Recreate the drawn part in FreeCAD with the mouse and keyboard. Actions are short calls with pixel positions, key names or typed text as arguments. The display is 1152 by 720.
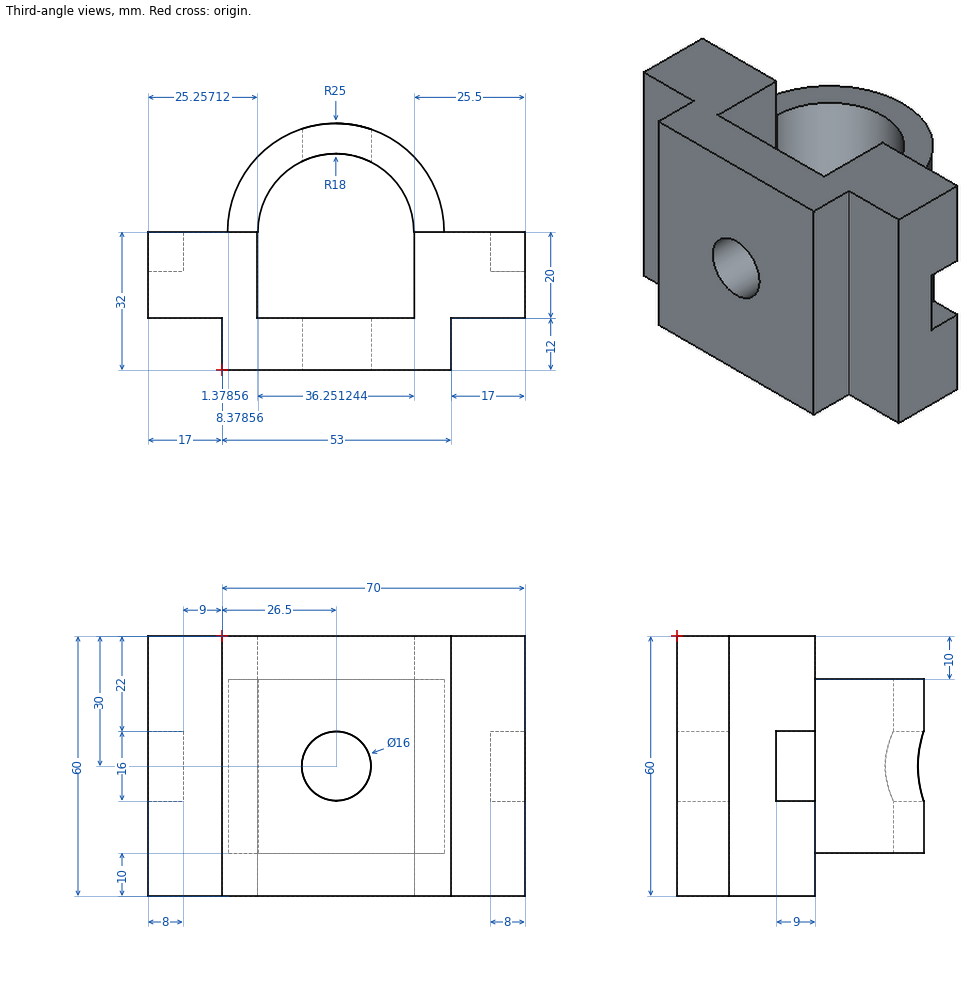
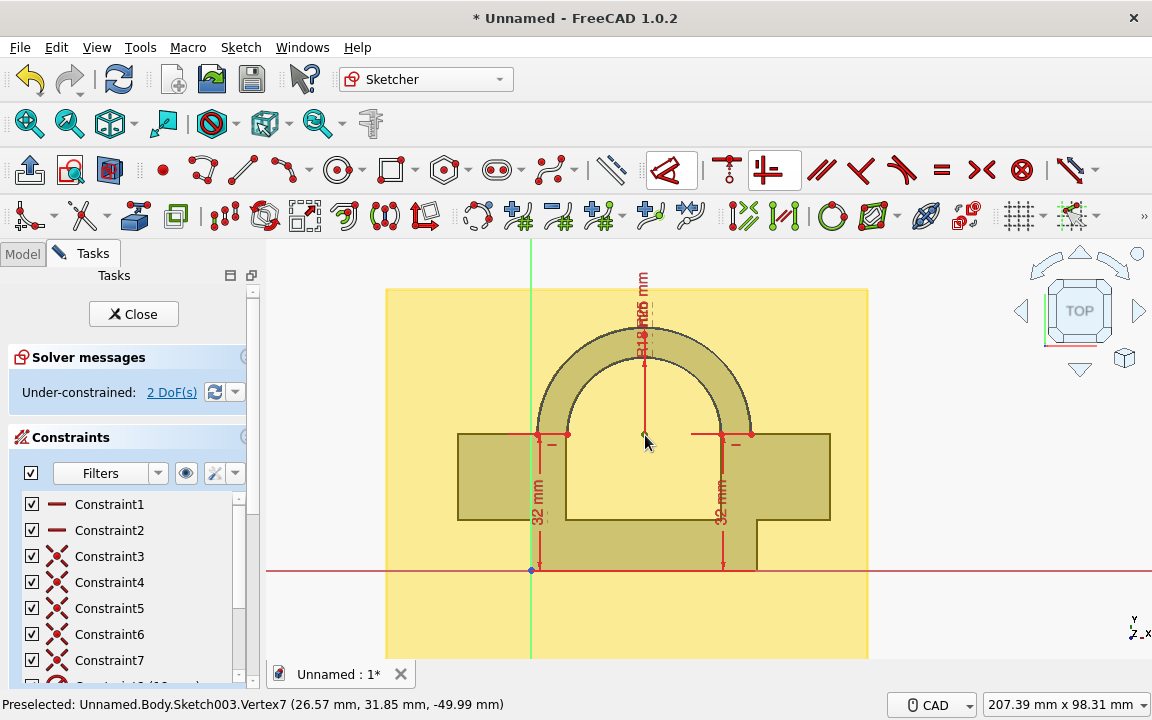
key(i)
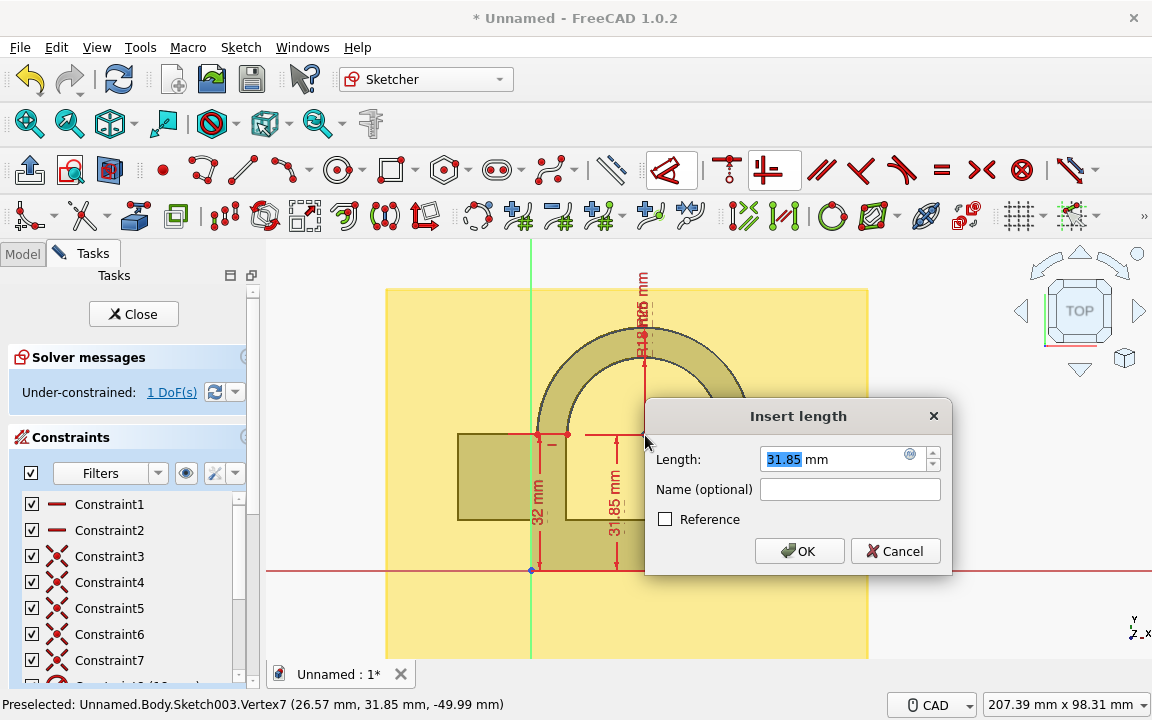
text(32)
key(Return)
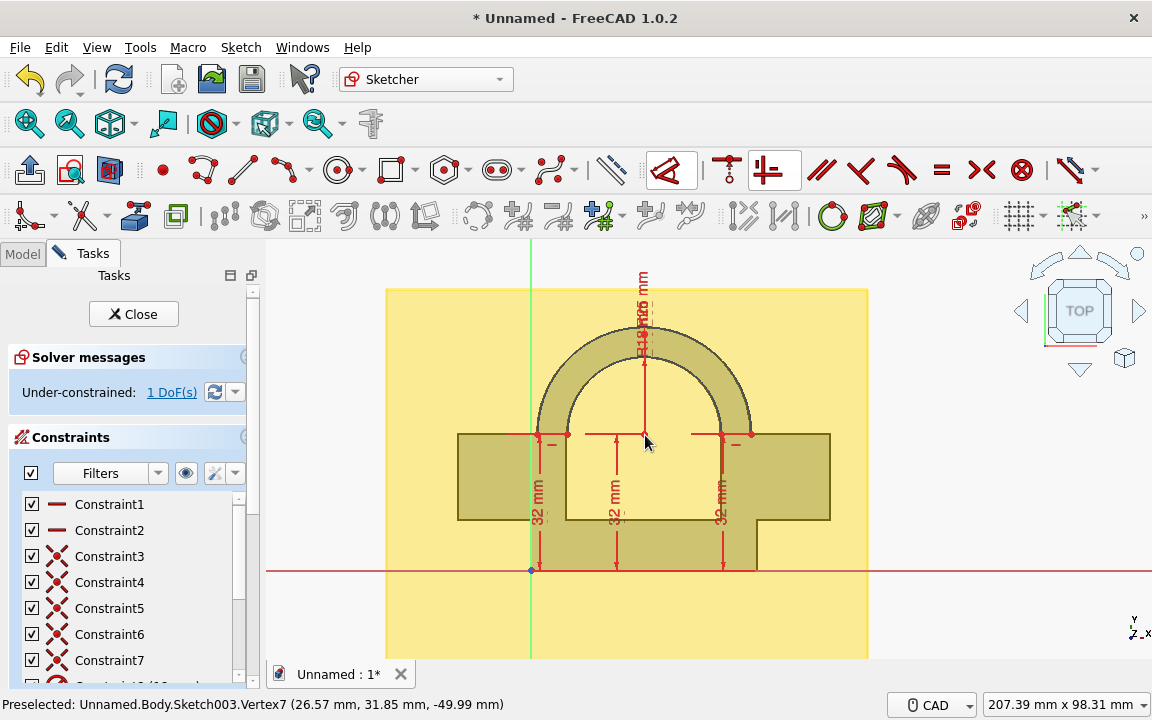
click(568, 434)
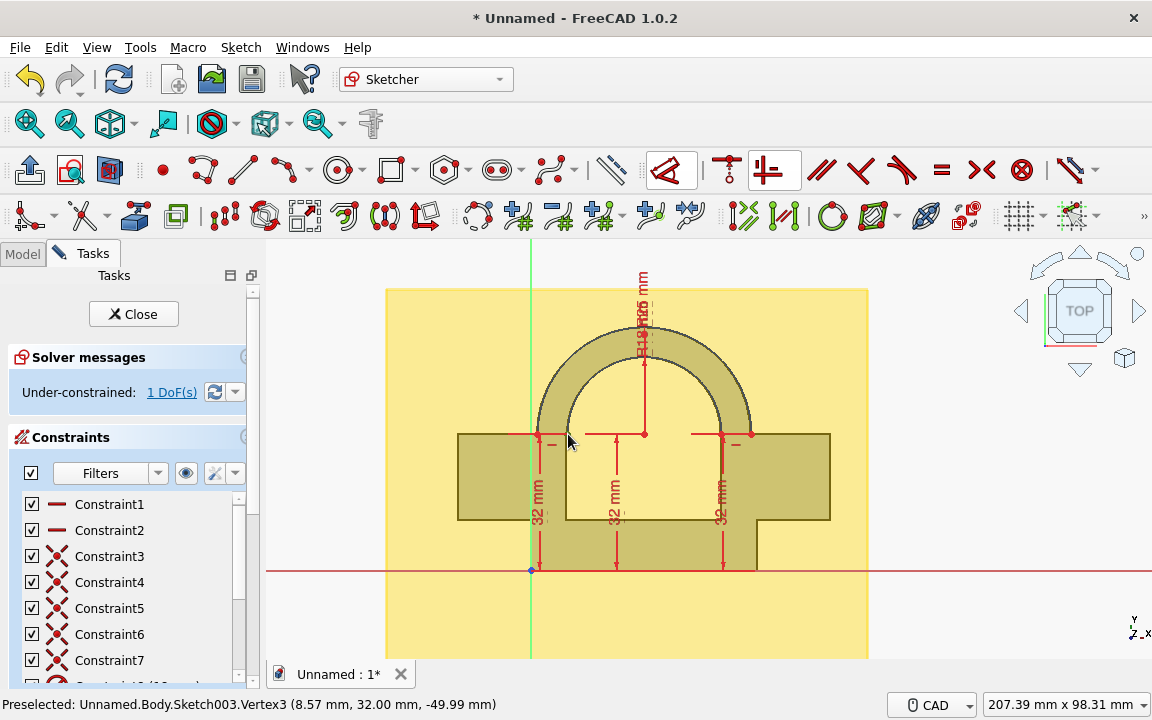
key(l)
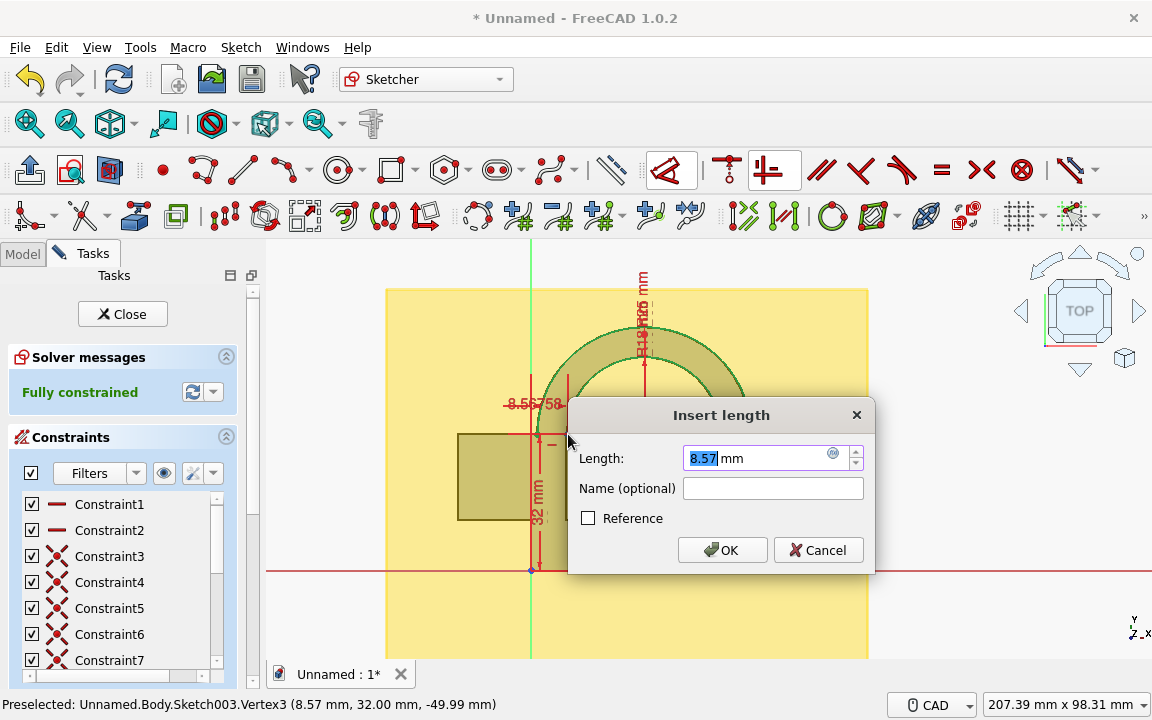
text(8.37856)
key(Return)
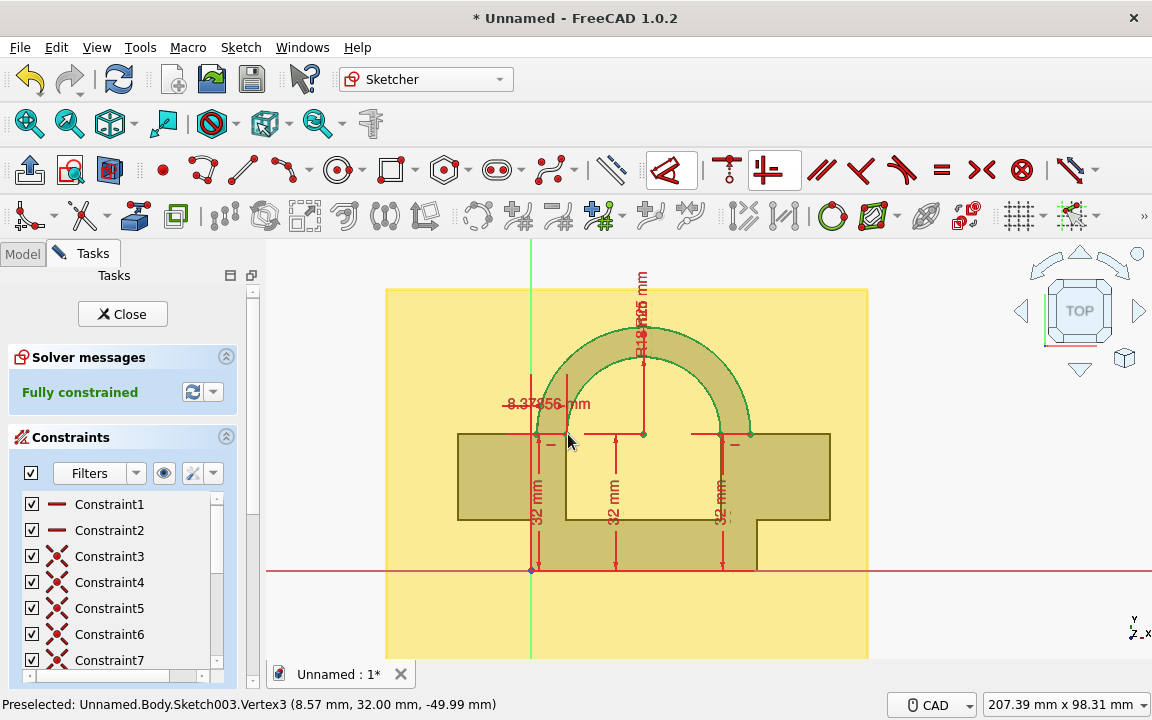
click(123, 314)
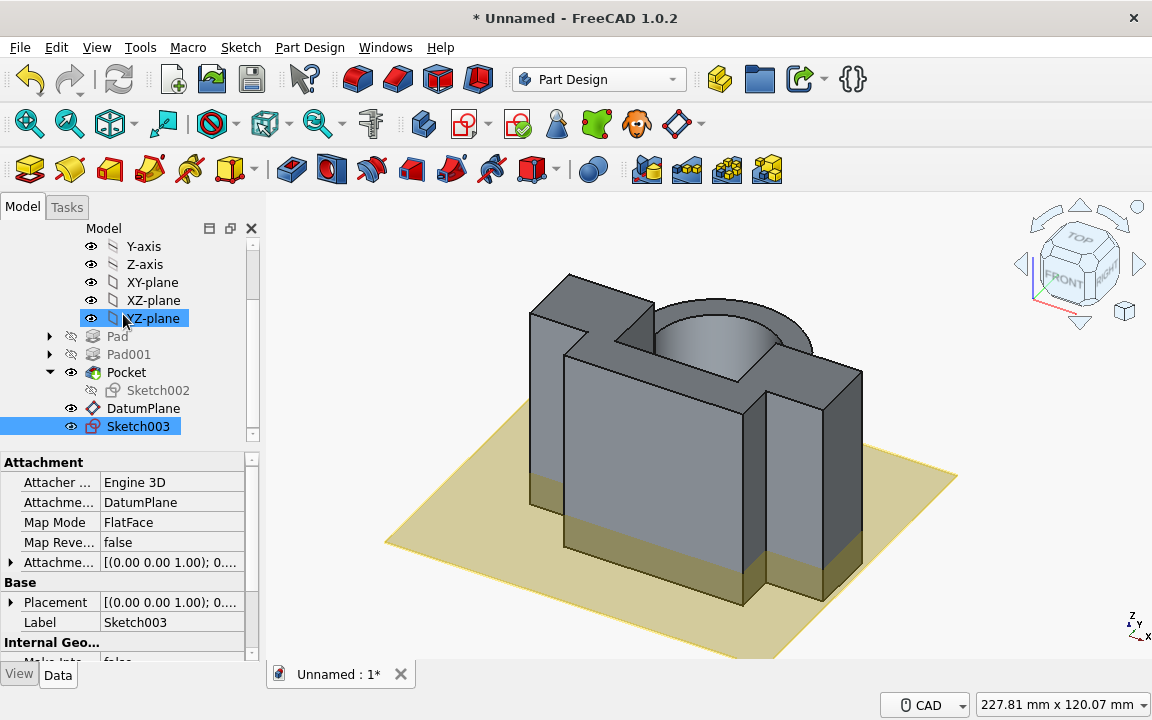
click(292, 170)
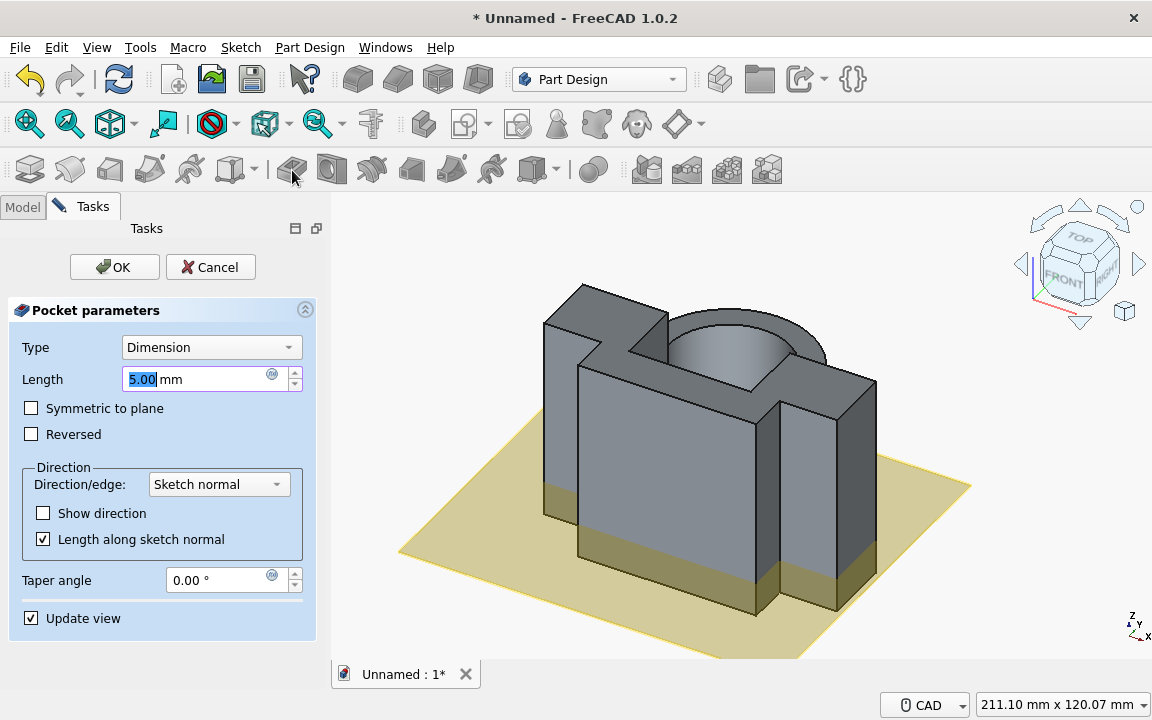
text(10)
key(Tab)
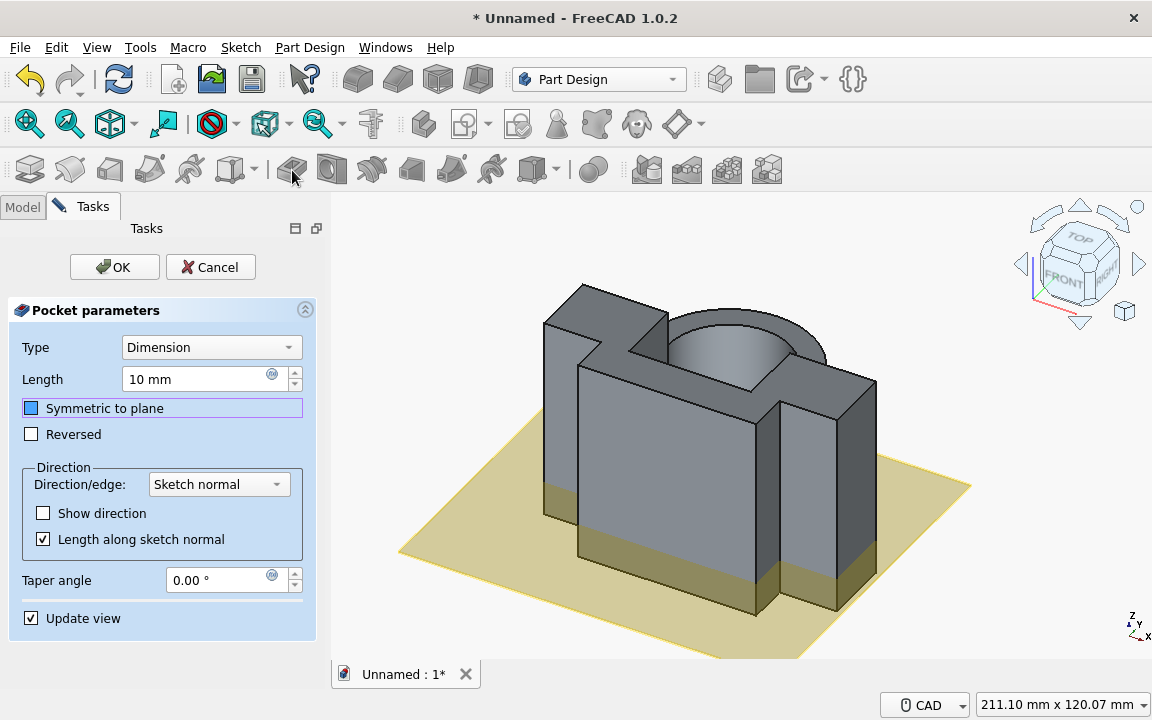
click(115, 267)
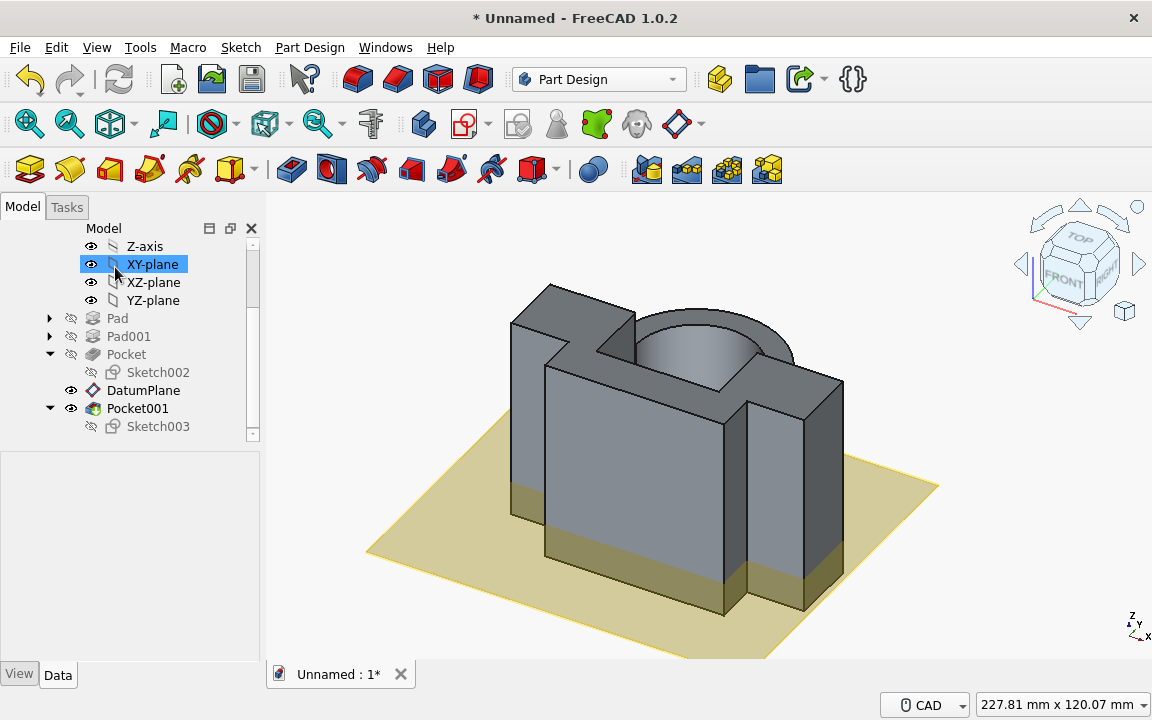
click(116, 390)
key(space)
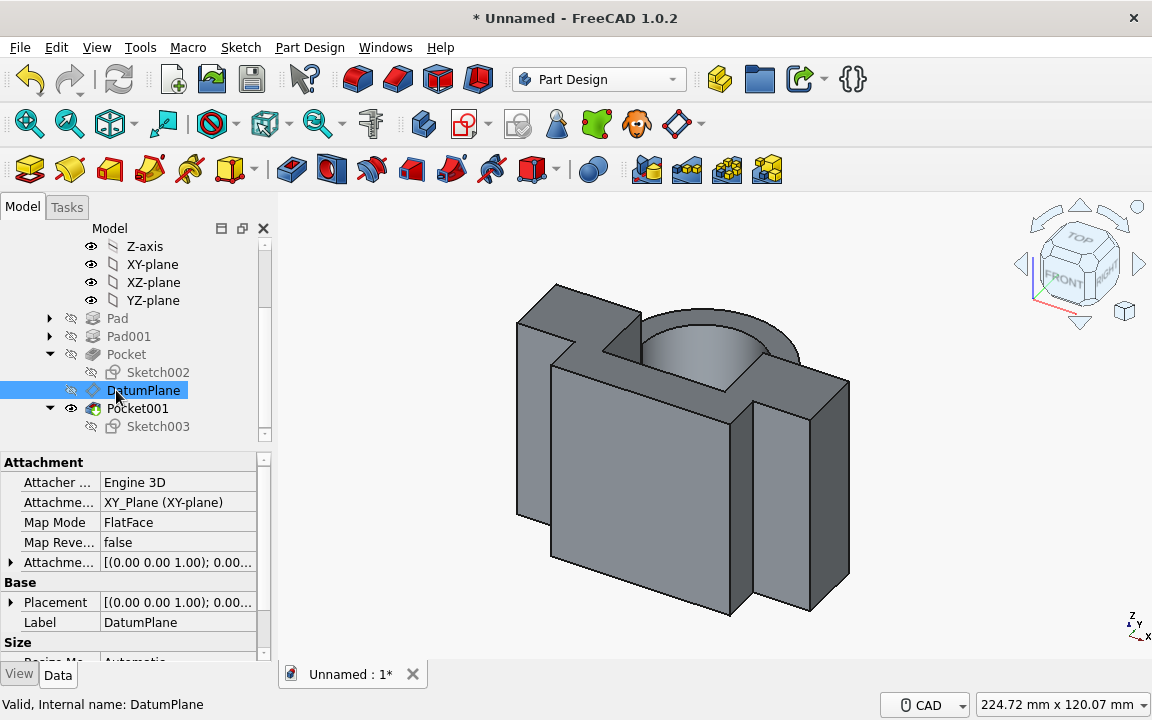
click(641, 489)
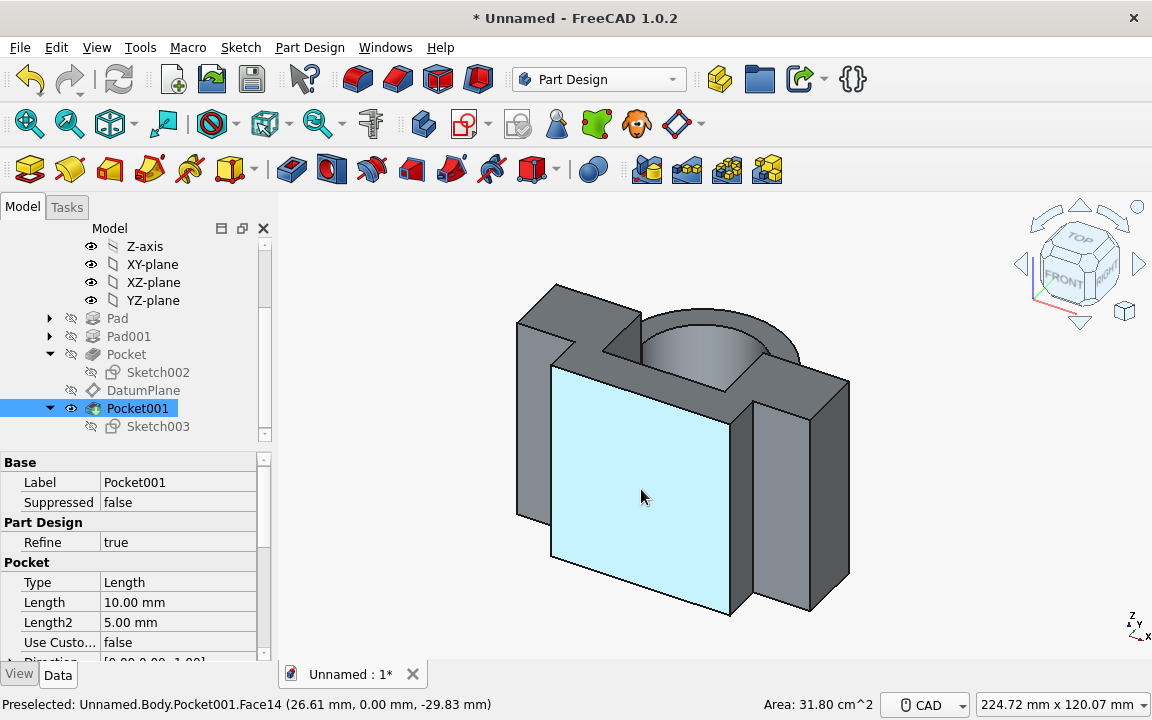
click(464, 124)